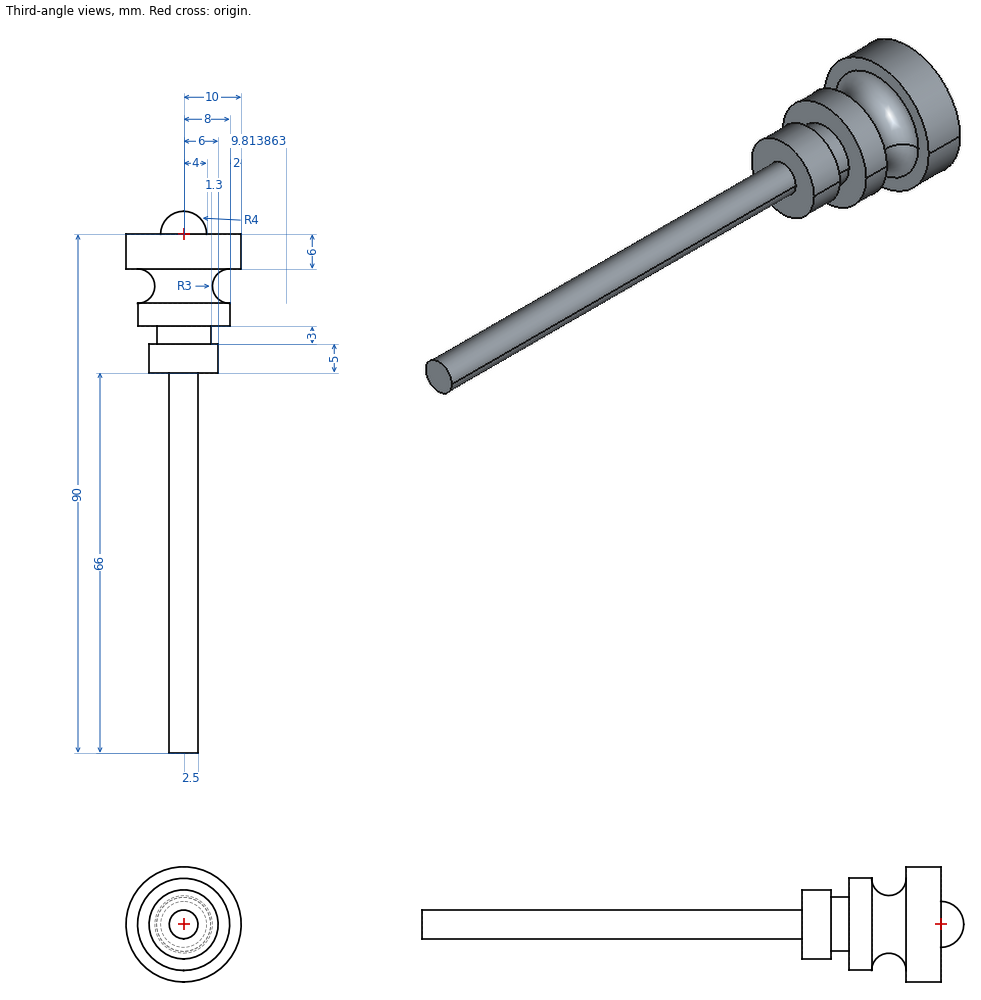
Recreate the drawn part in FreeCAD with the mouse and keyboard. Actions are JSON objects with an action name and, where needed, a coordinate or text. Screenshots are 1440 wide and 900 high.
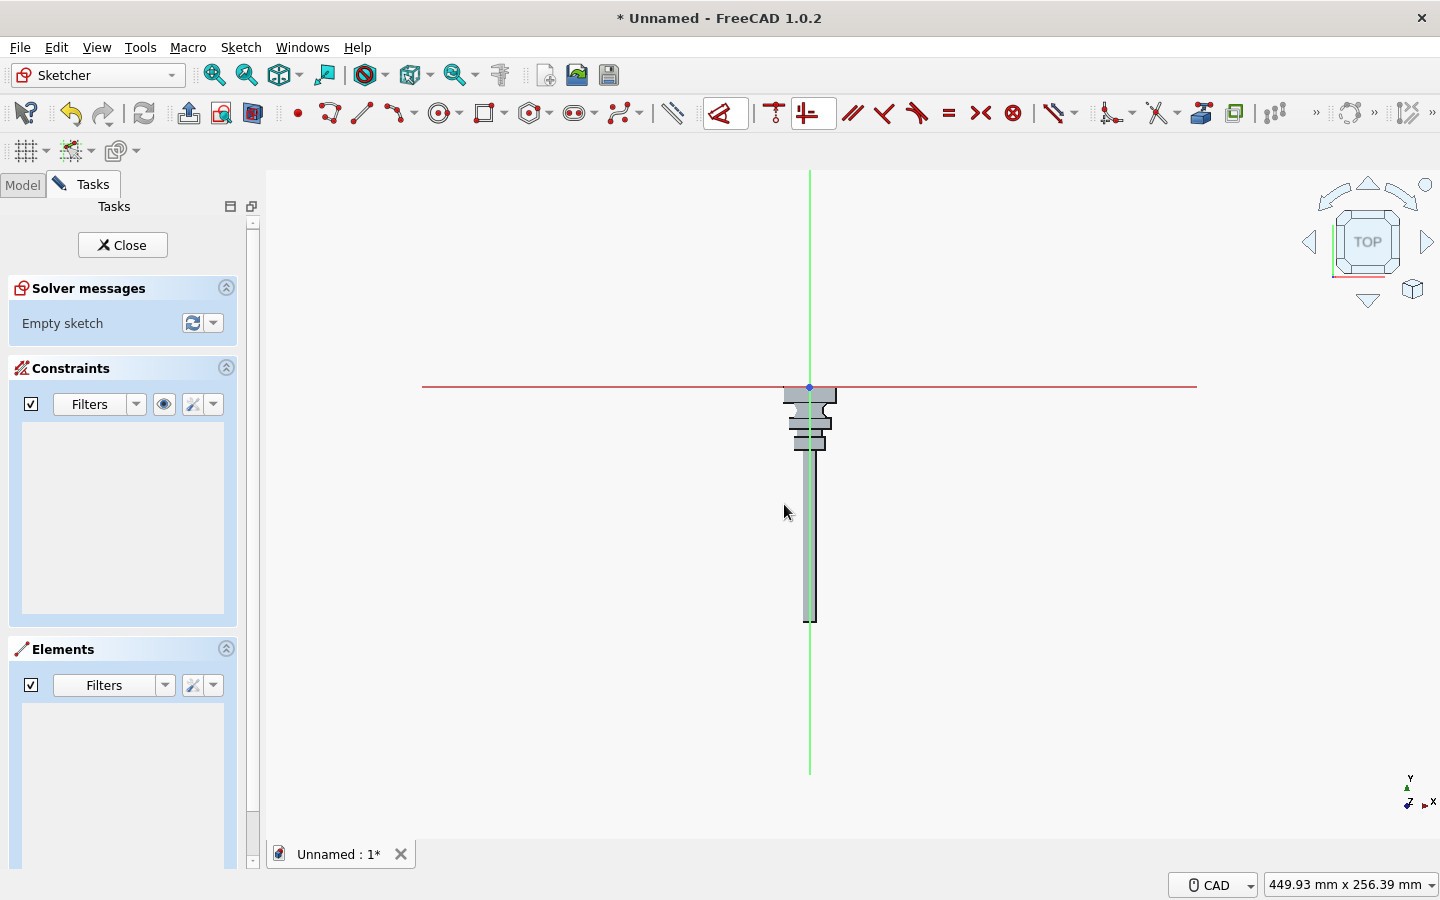
{"action": "scroll", "coordinate": [816, 375], "scroll_direction": "up", "scroll_amount": 15}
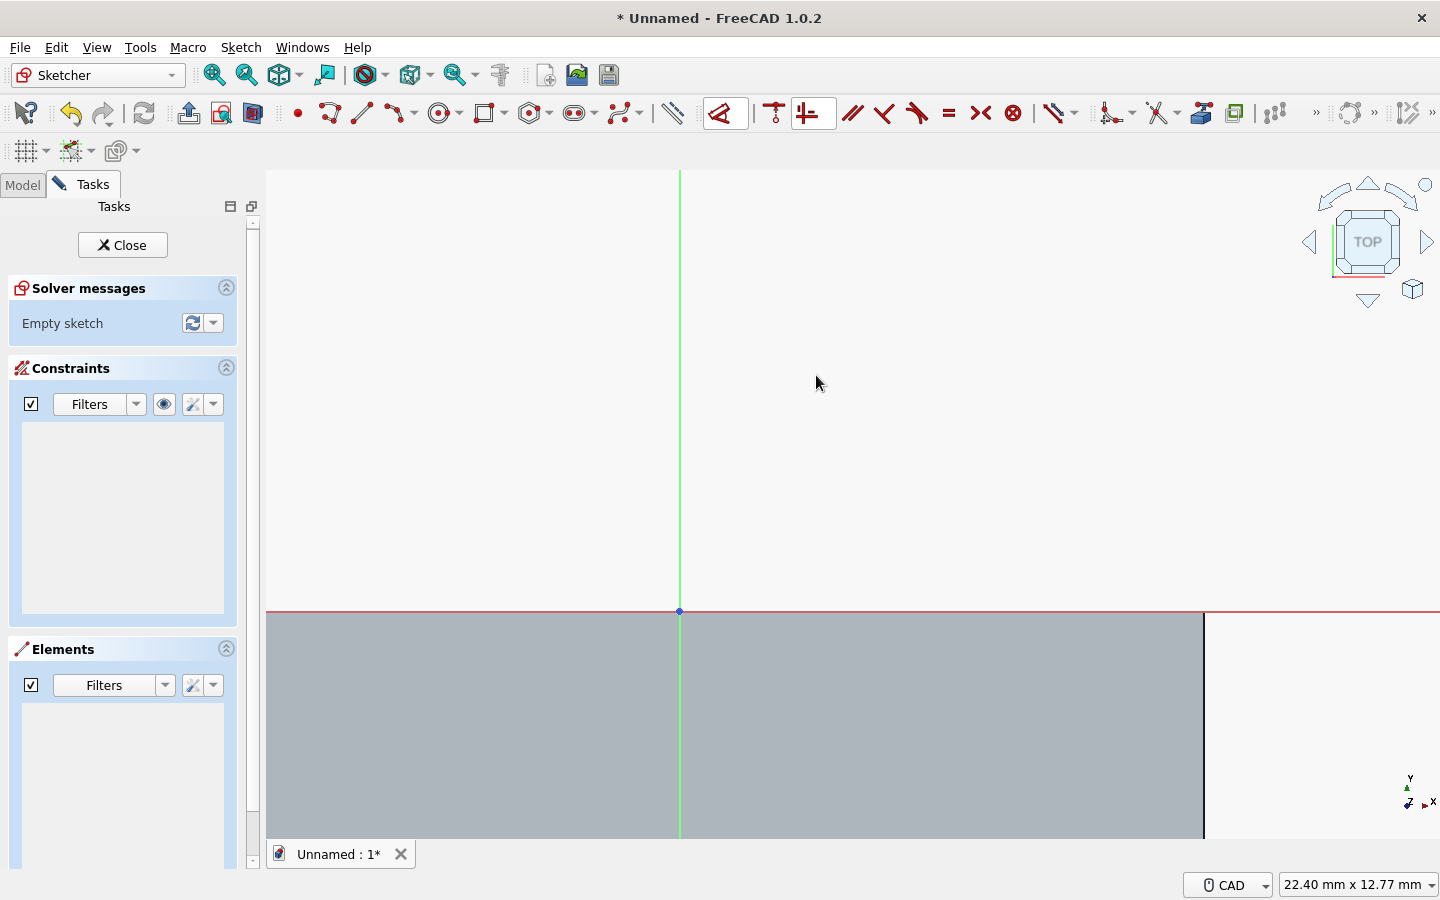
{"action": "scroll", "coordinate": [785, 509], "scroll_direction": "up", "scroll_amount": 4}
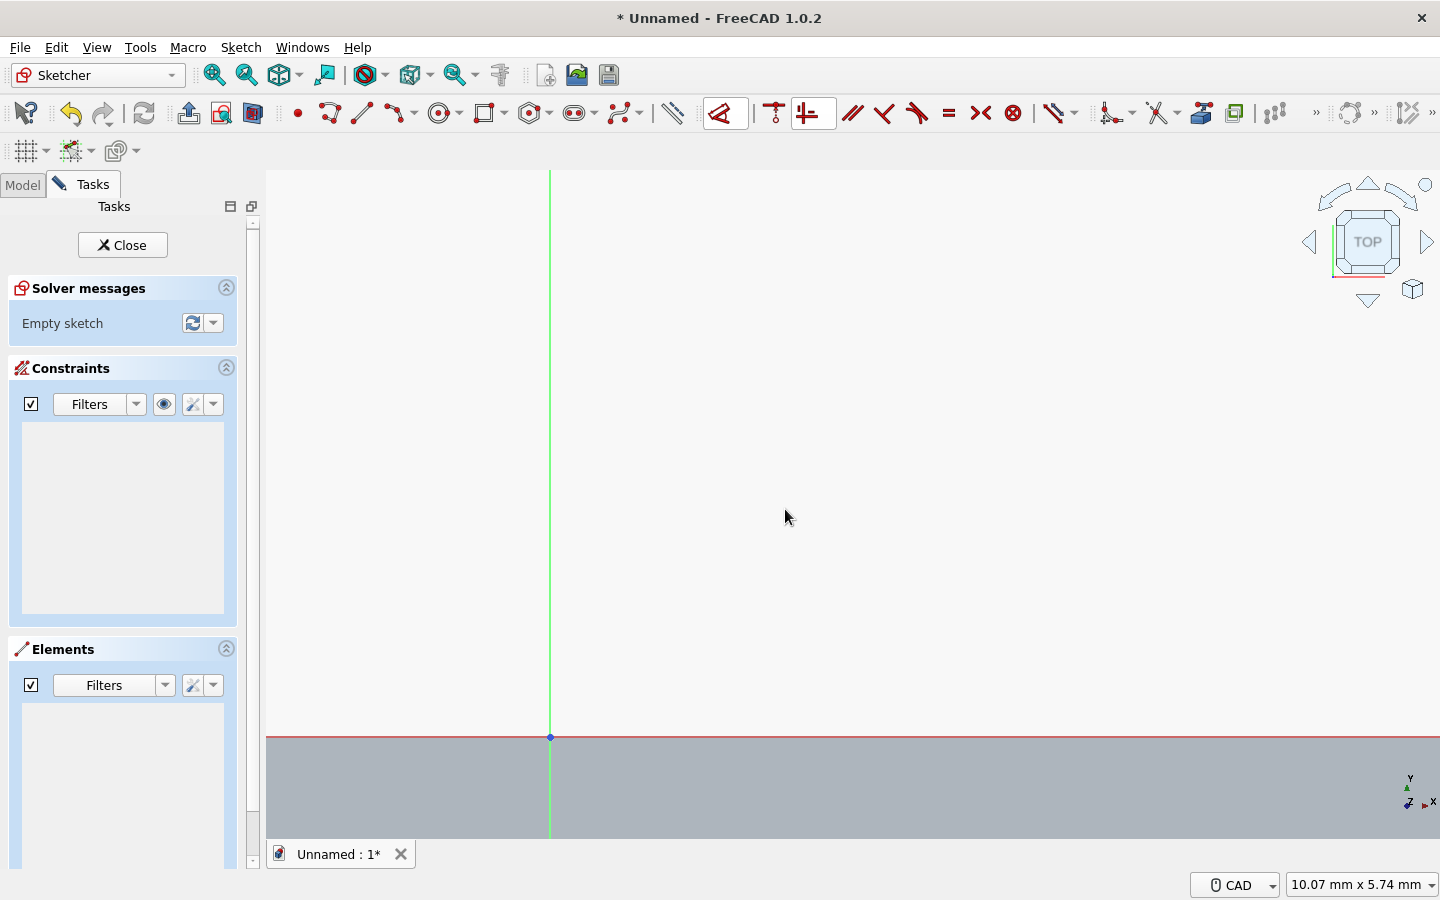
{"action": "left_click", "coordinate": [330, 114]}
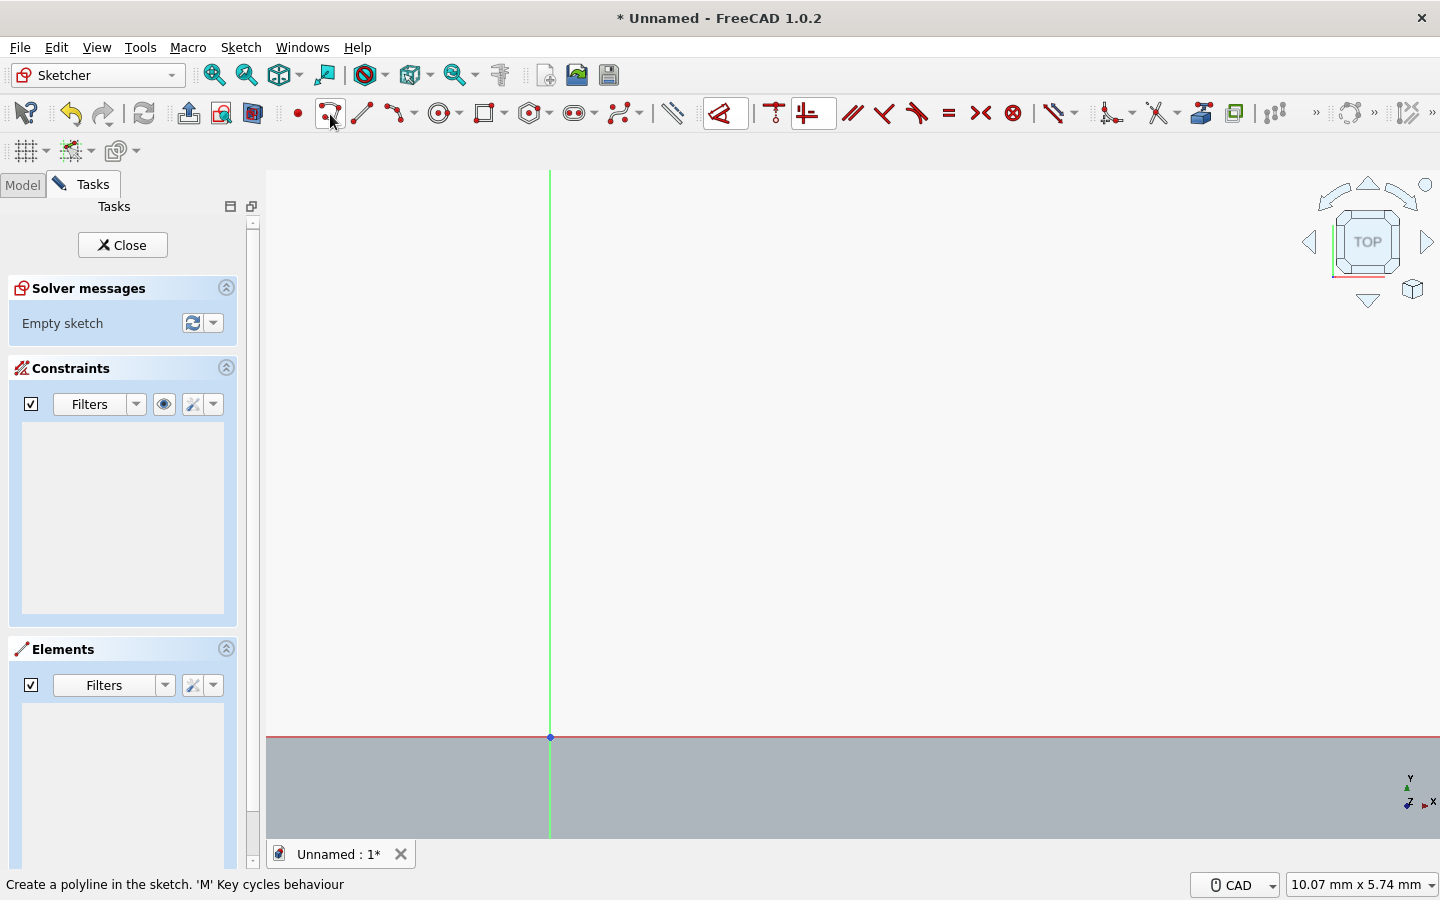
{"action": "left_click", "coordinate": [550, 271]}
{"action": "left_click", "coordinate": [550, 737]}
{"action": "left_click", "coordinate": [1017, 728]}
{"action": "right_click", "coordinate": [1017, 728]}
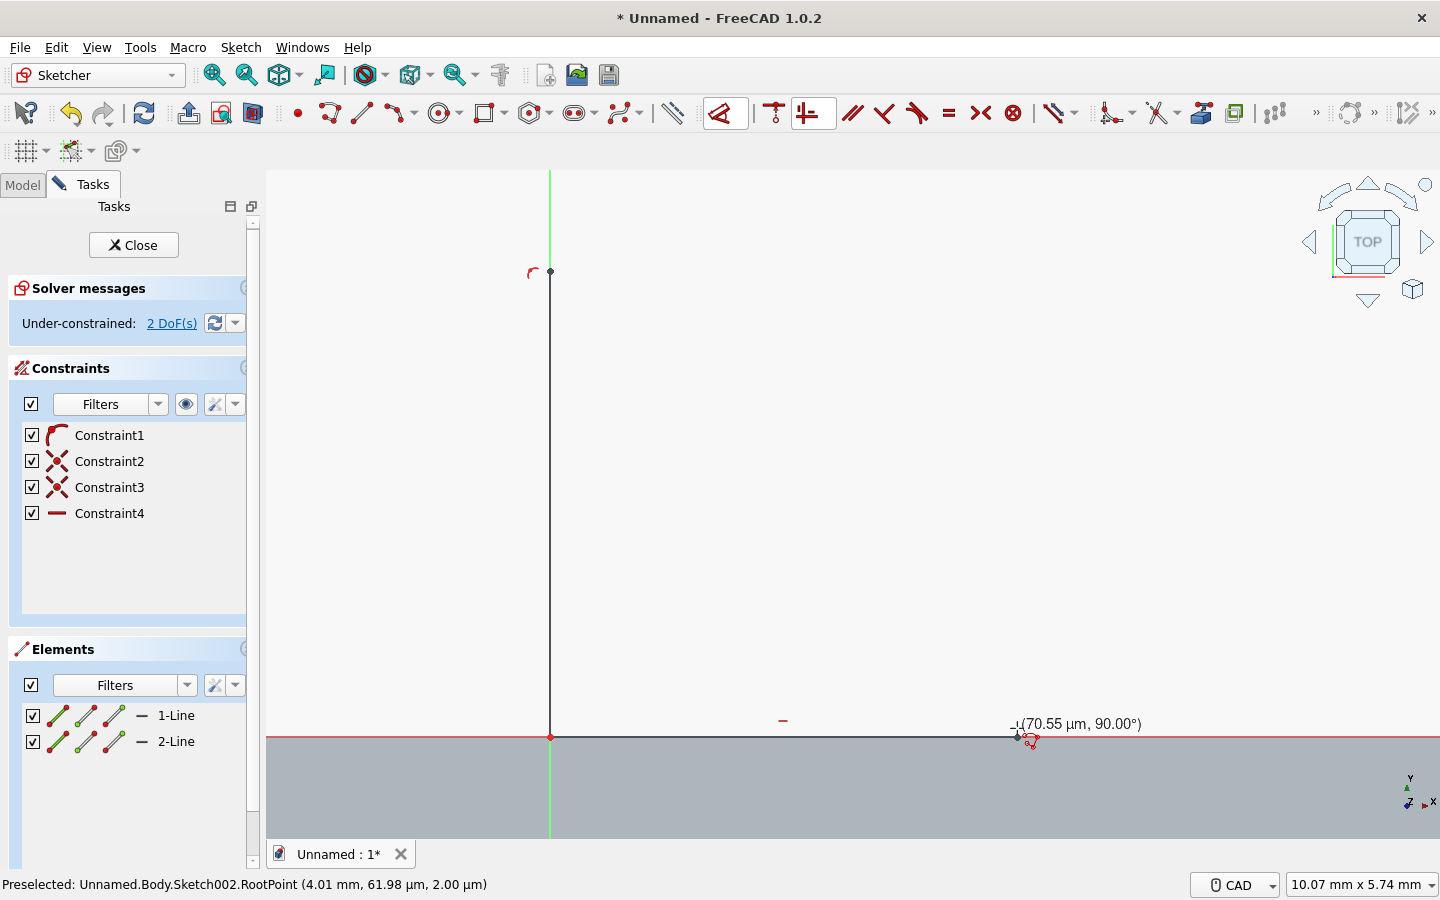
{"action": "key", "text": "g 3 a"}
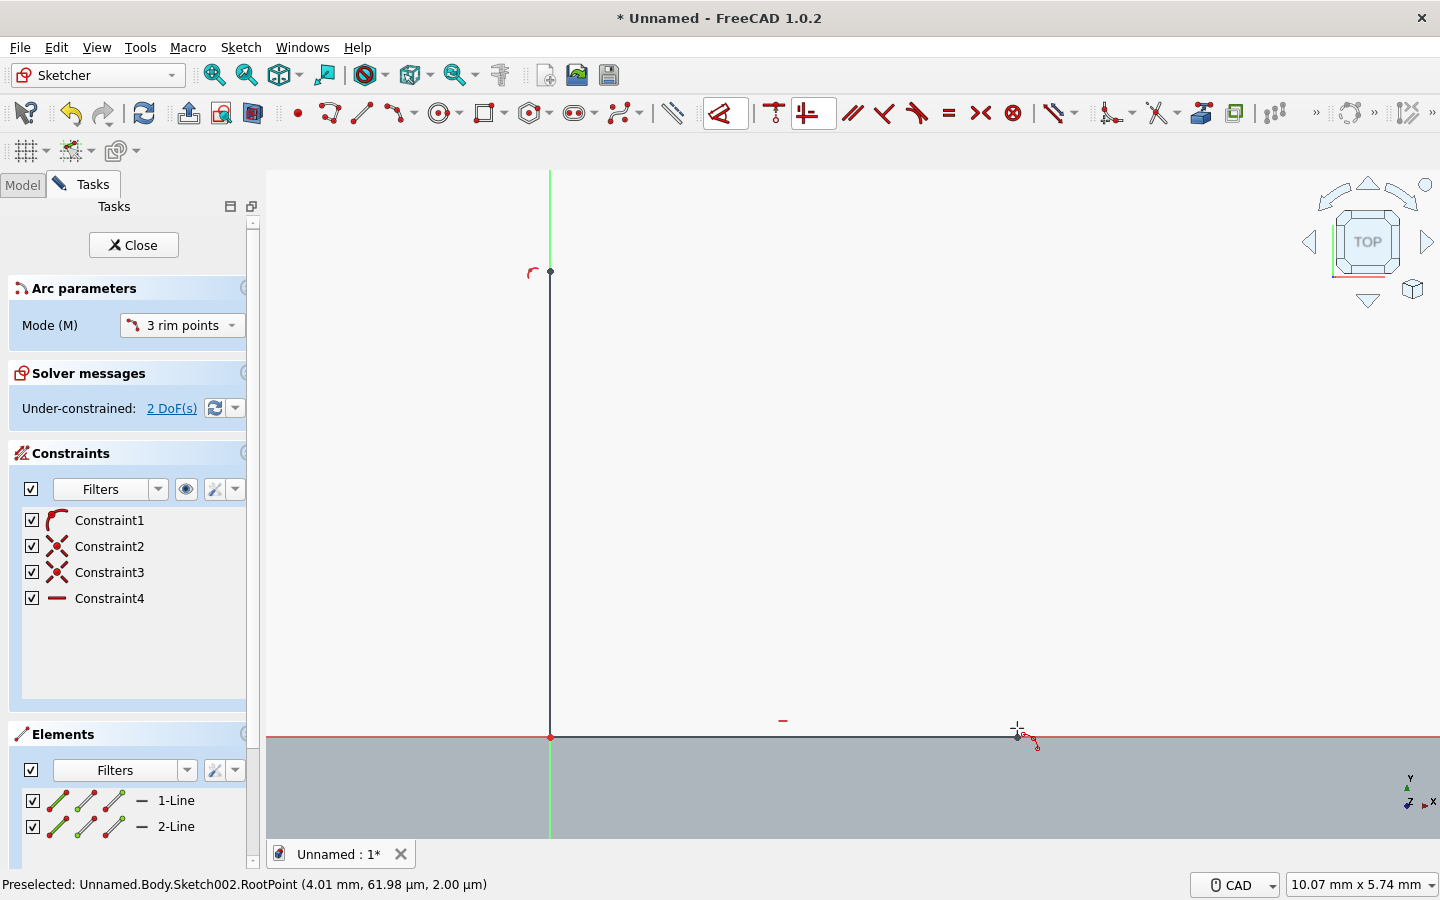
{"action": "left_click", "coordinate": [1017, 728]}
{"action": "left_click", "coordinate": [550, 272]}
{"action": "left_click", "coordinate": [880, 407]}
{"action": "key", "text": "Escape"}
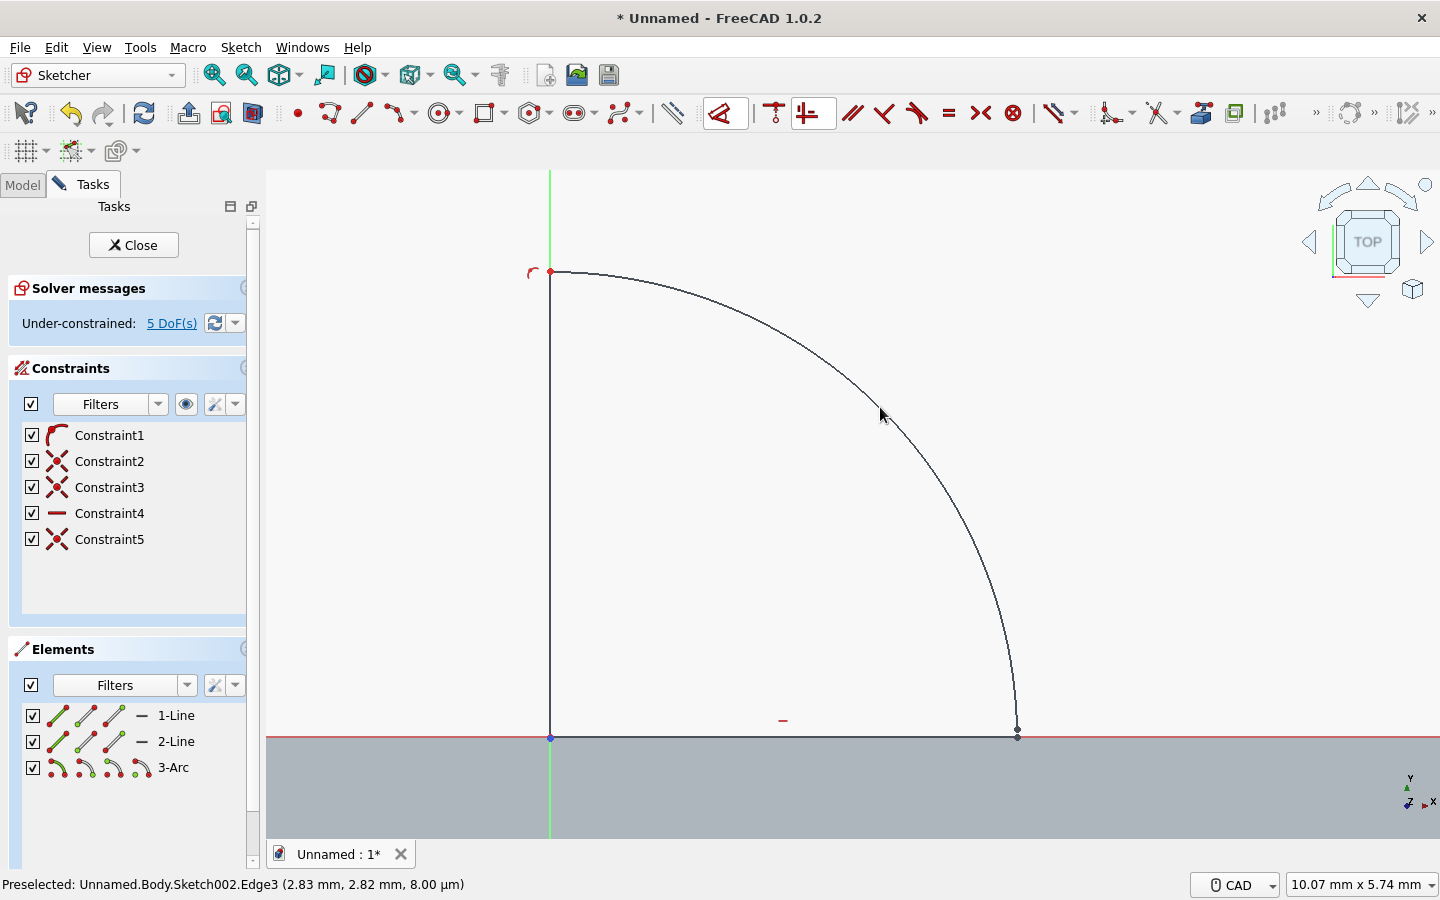
{"action": "scroll", "coordinate": [551, 738], "scroll_direction": "up", "scroll_amount": 22}